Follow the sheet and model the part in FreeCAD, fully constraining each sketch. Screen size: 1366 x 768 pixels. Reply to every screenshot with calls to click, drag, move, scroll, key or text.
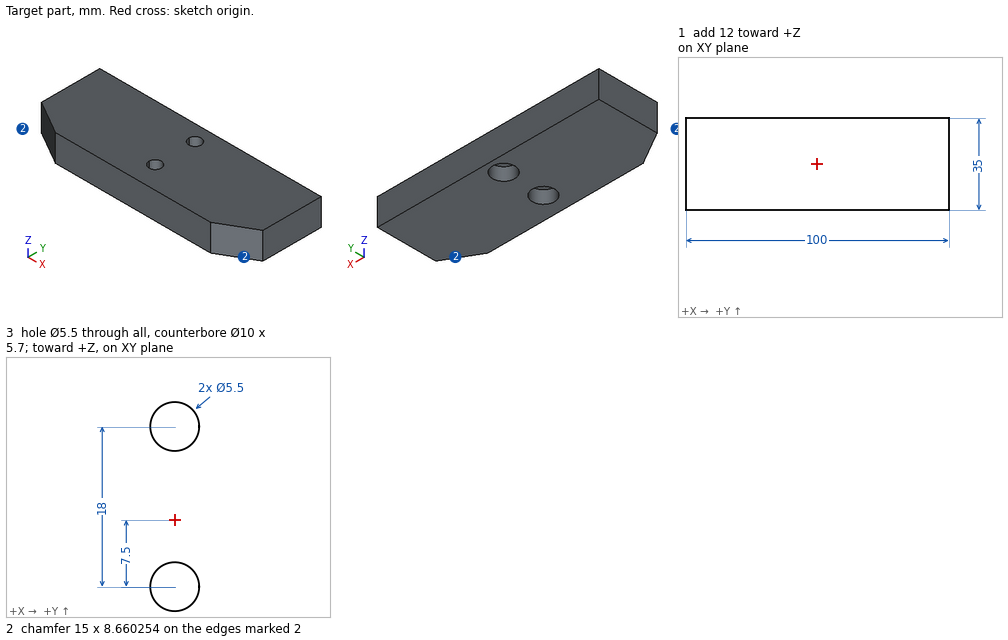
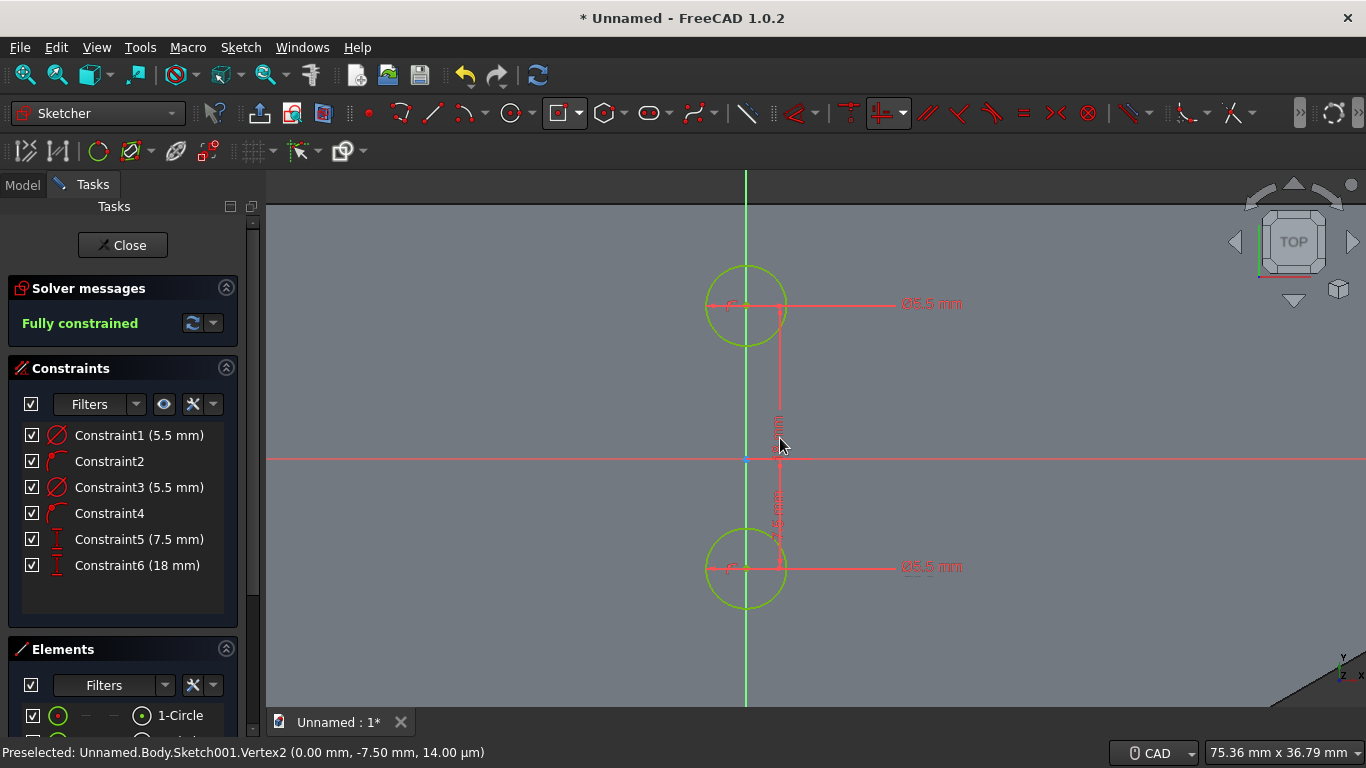
click(123, 245)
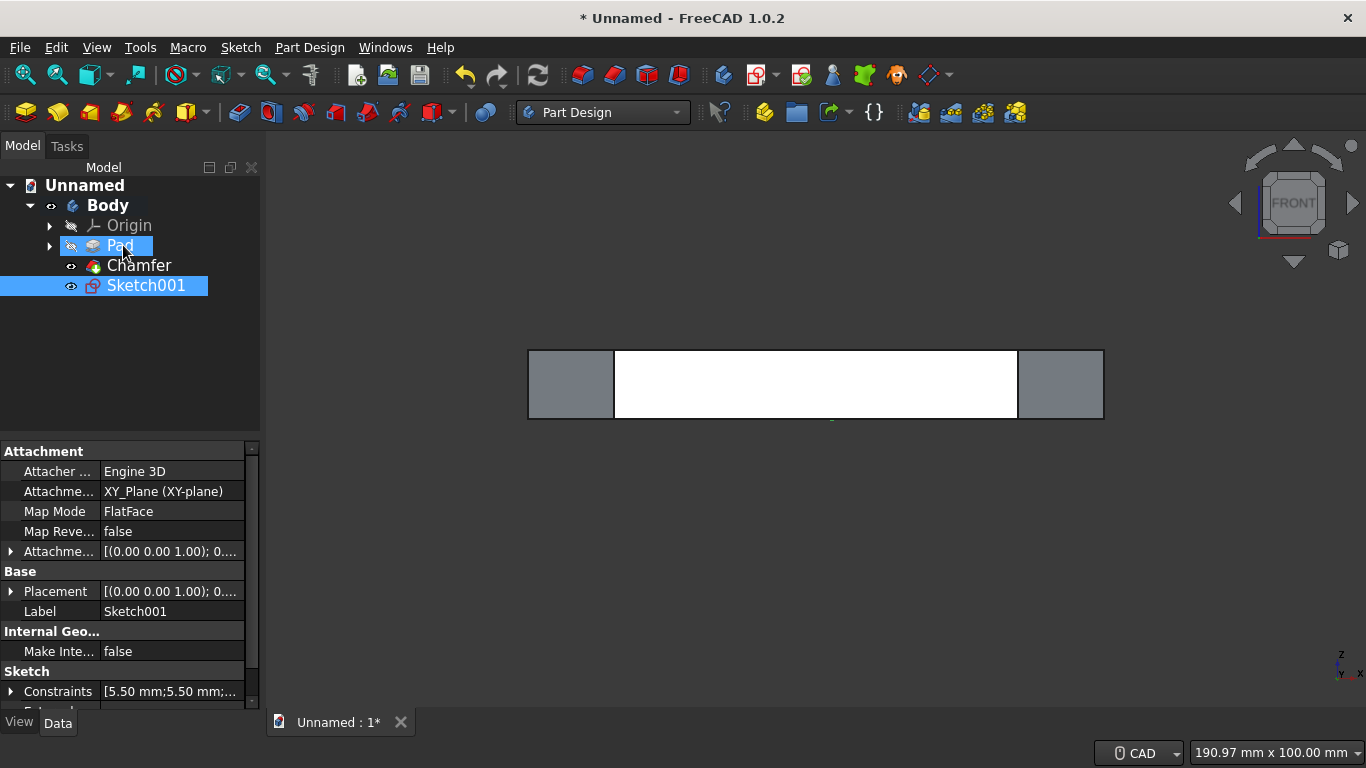
click(272, 112)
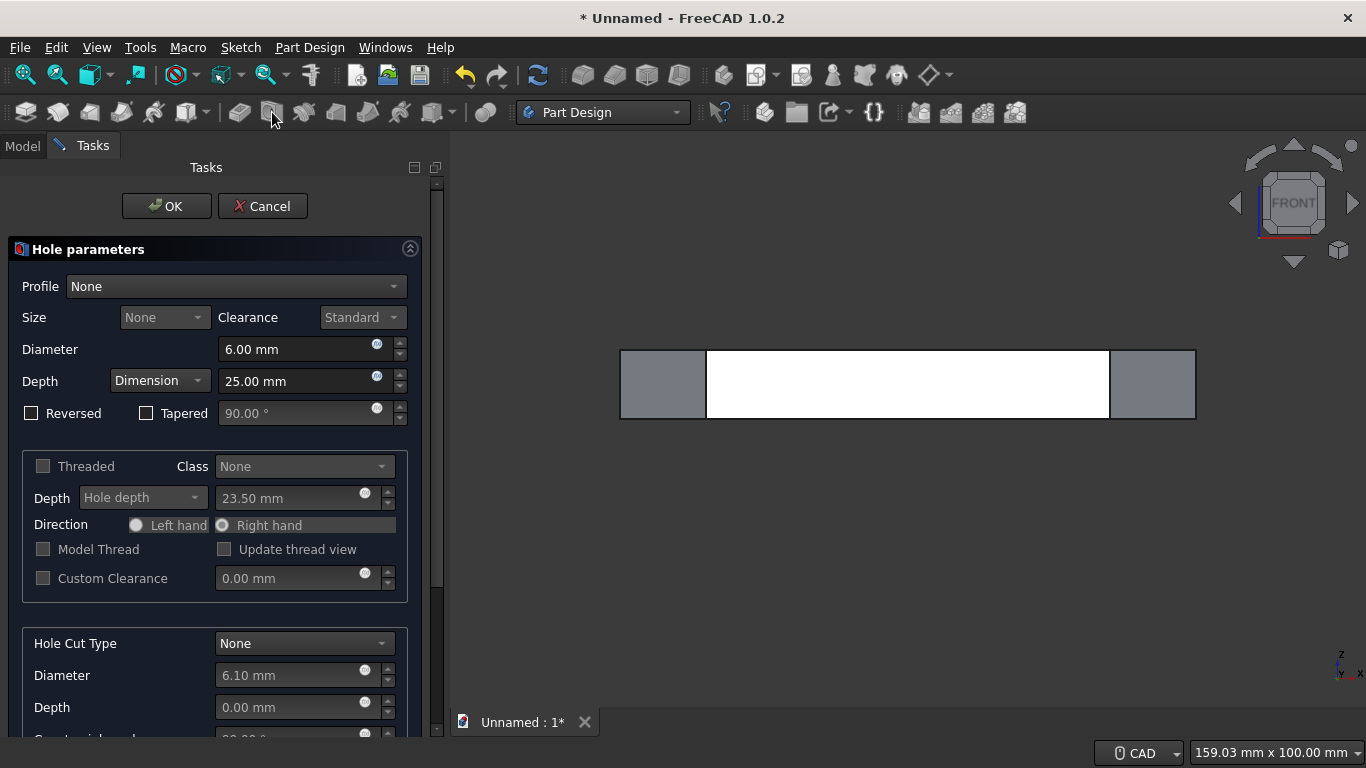
triple_click(305, 349)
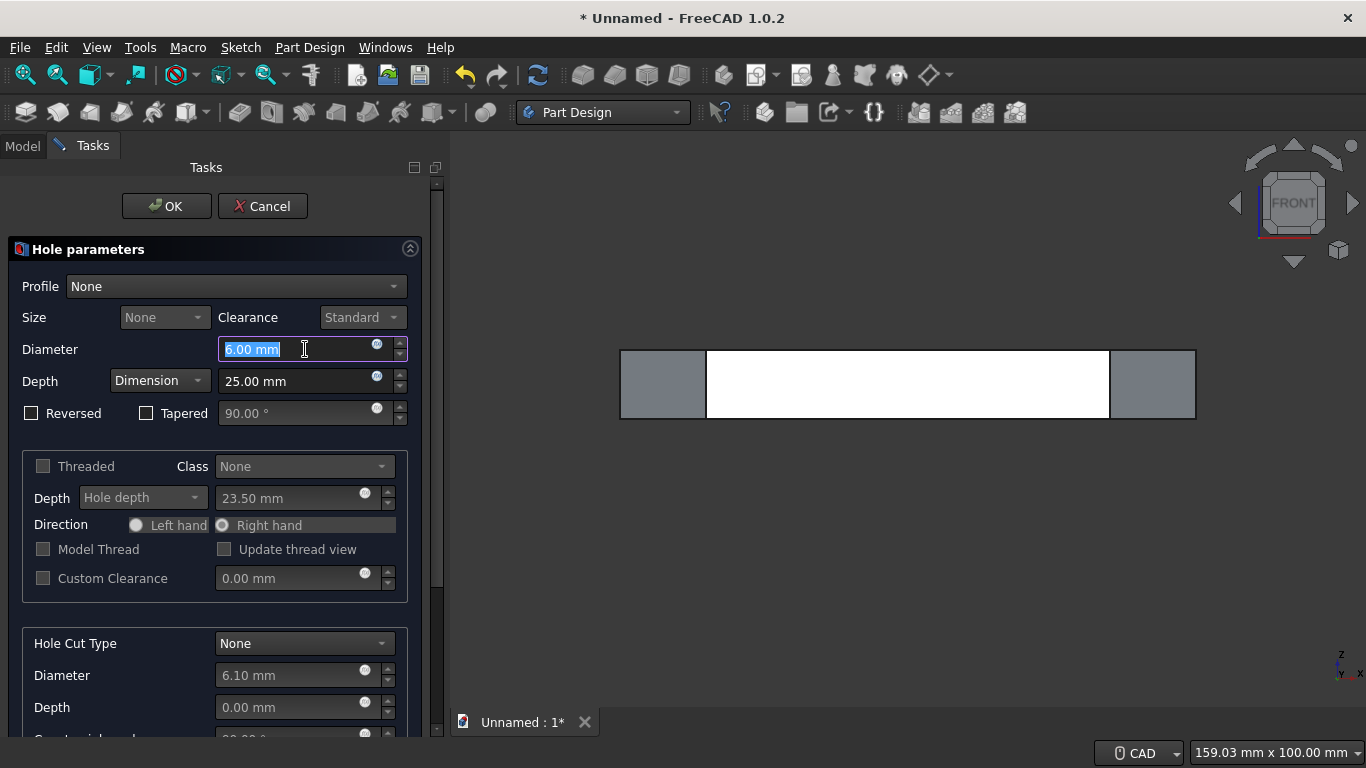
text(5.5)
key(Tab)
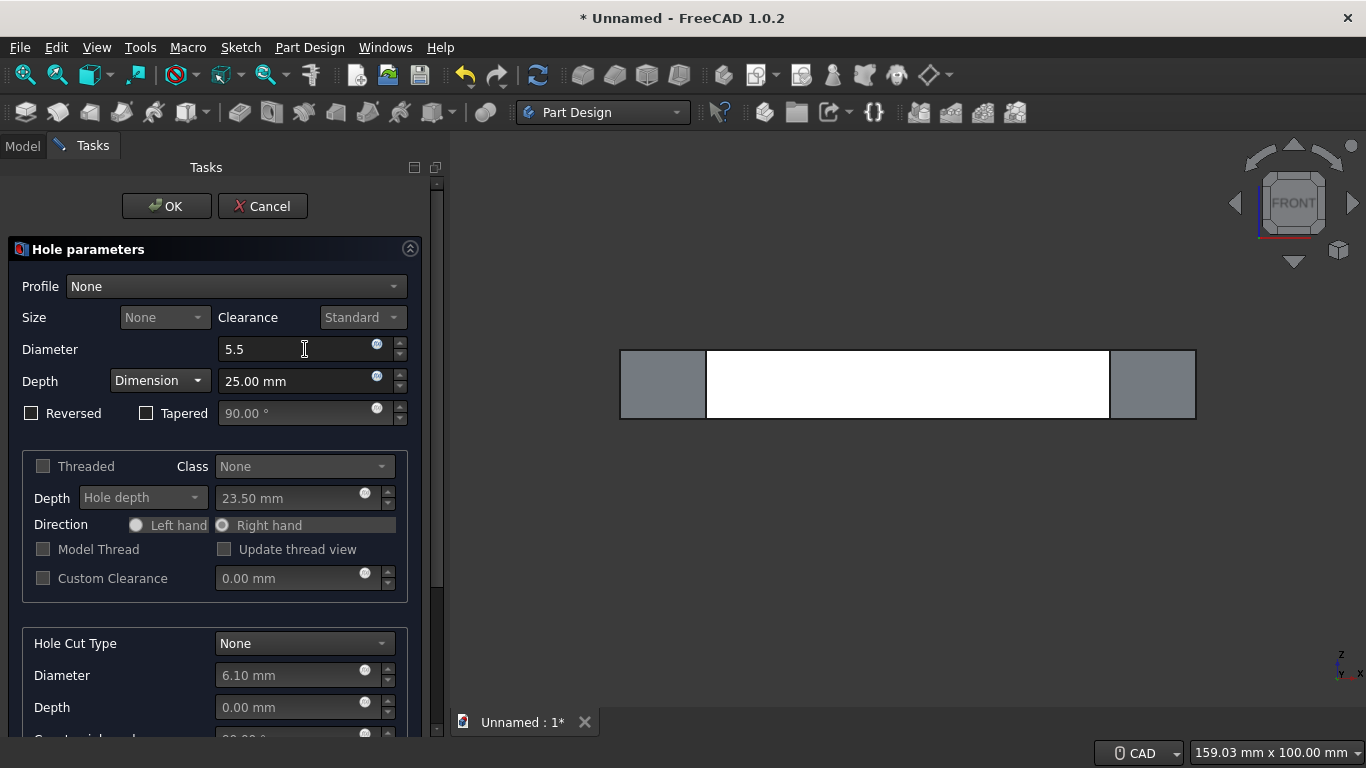
click(161, 380)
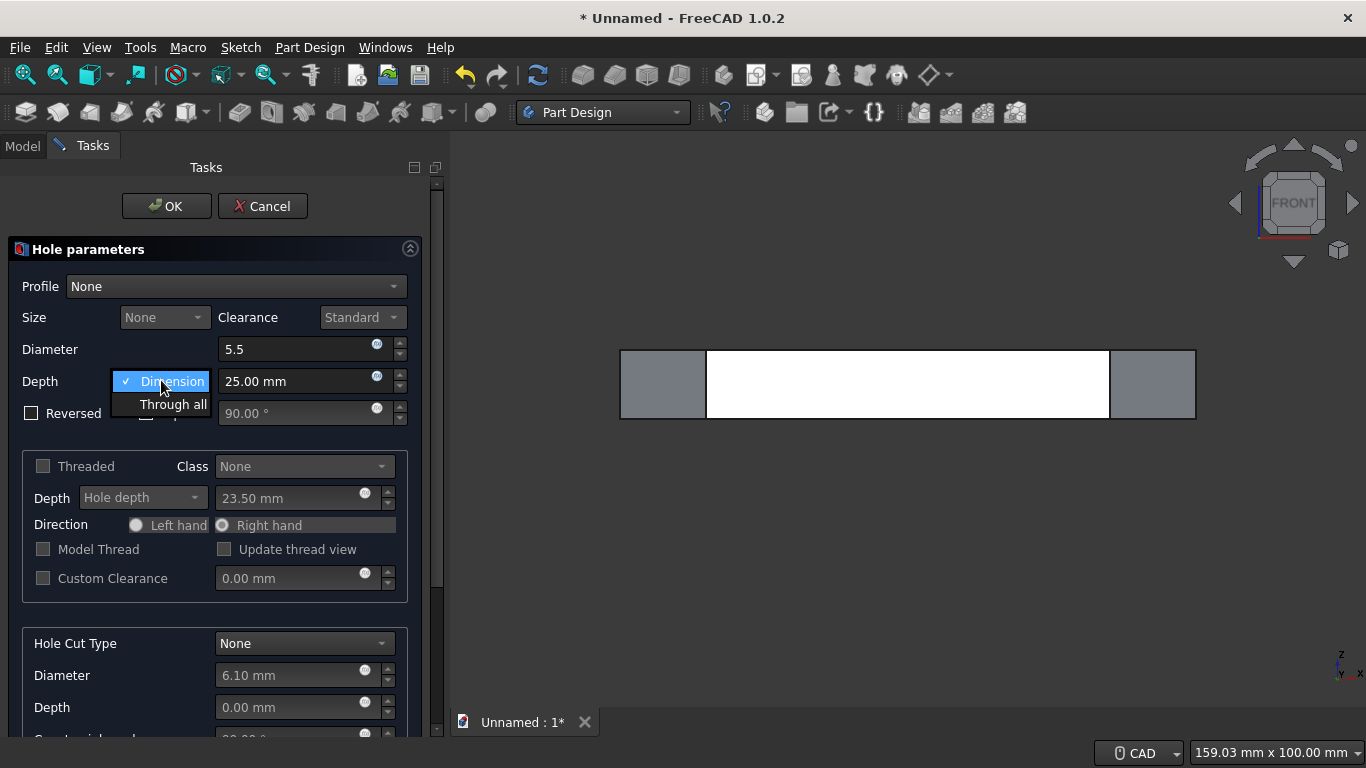
click(160, 404)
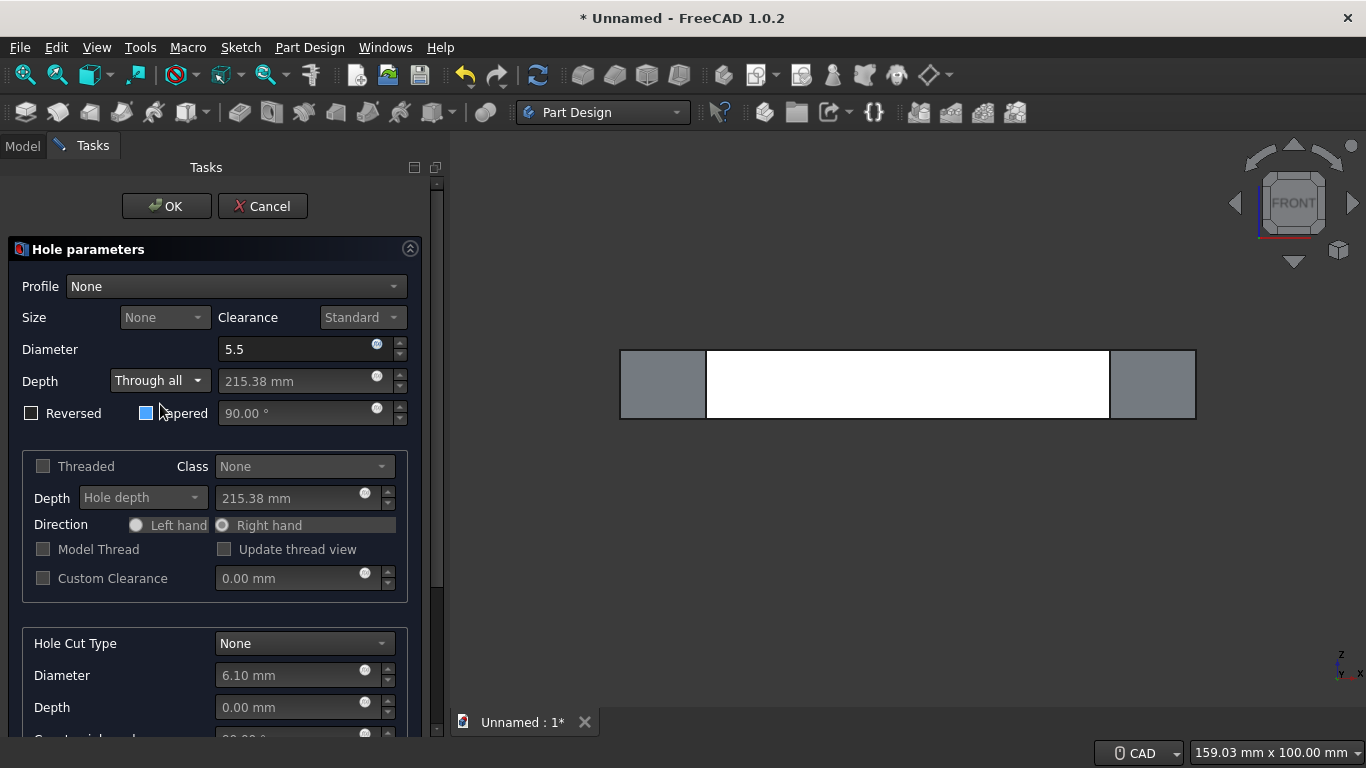
click(30, 413)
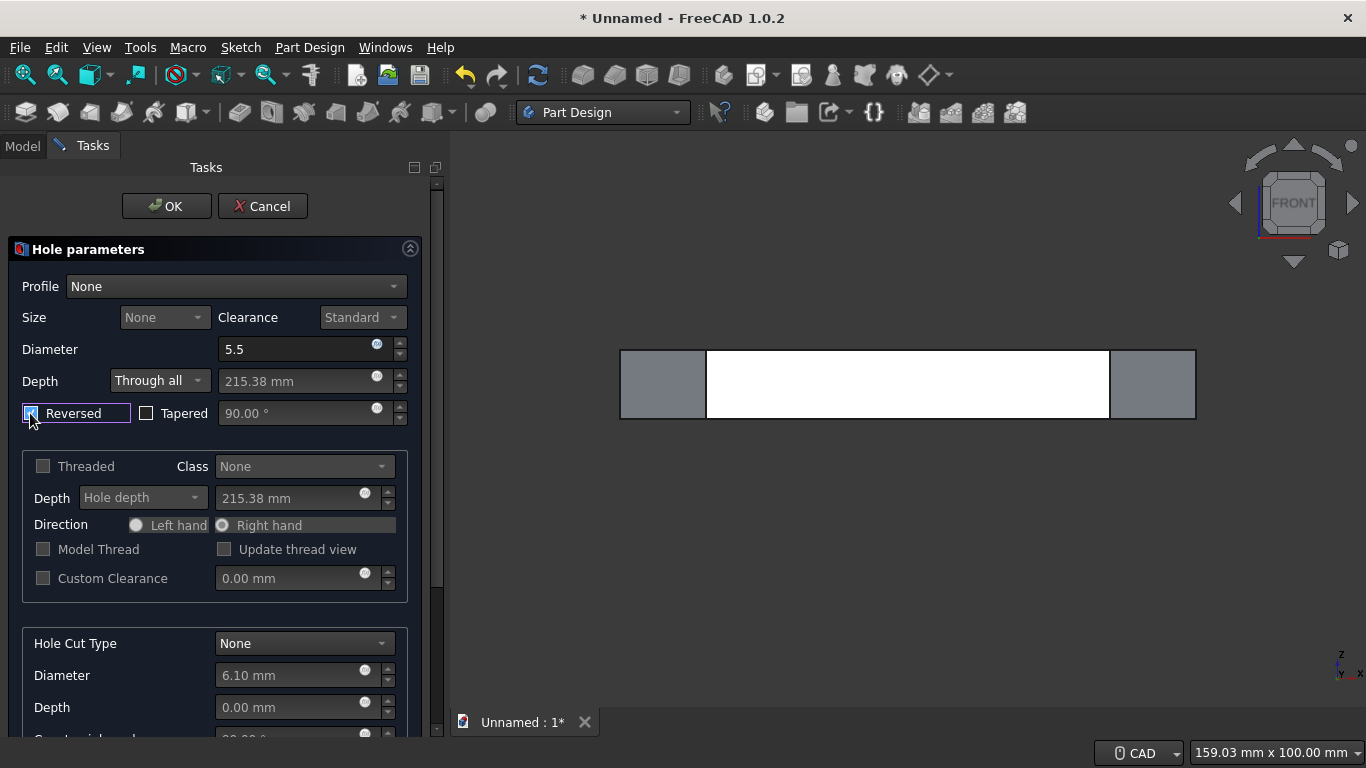
click(306, 644)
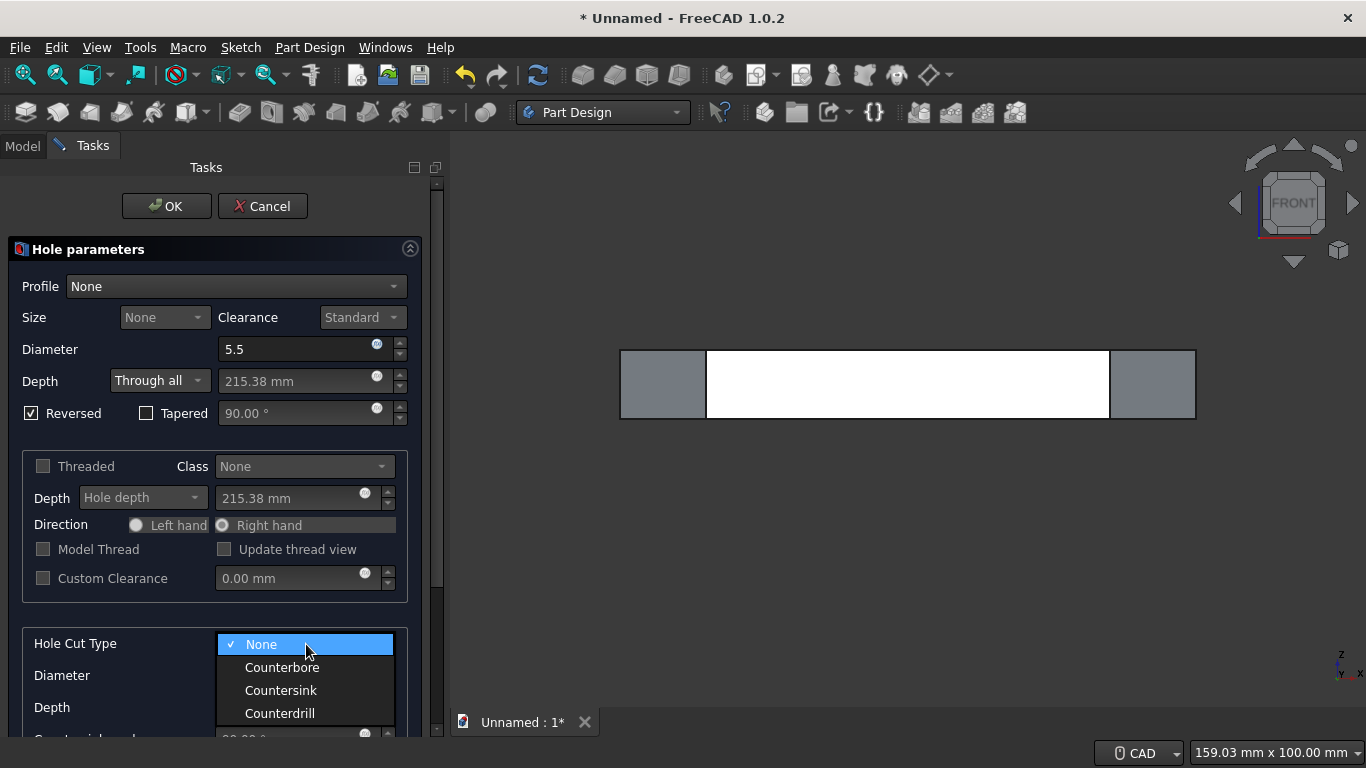
click(304, 668)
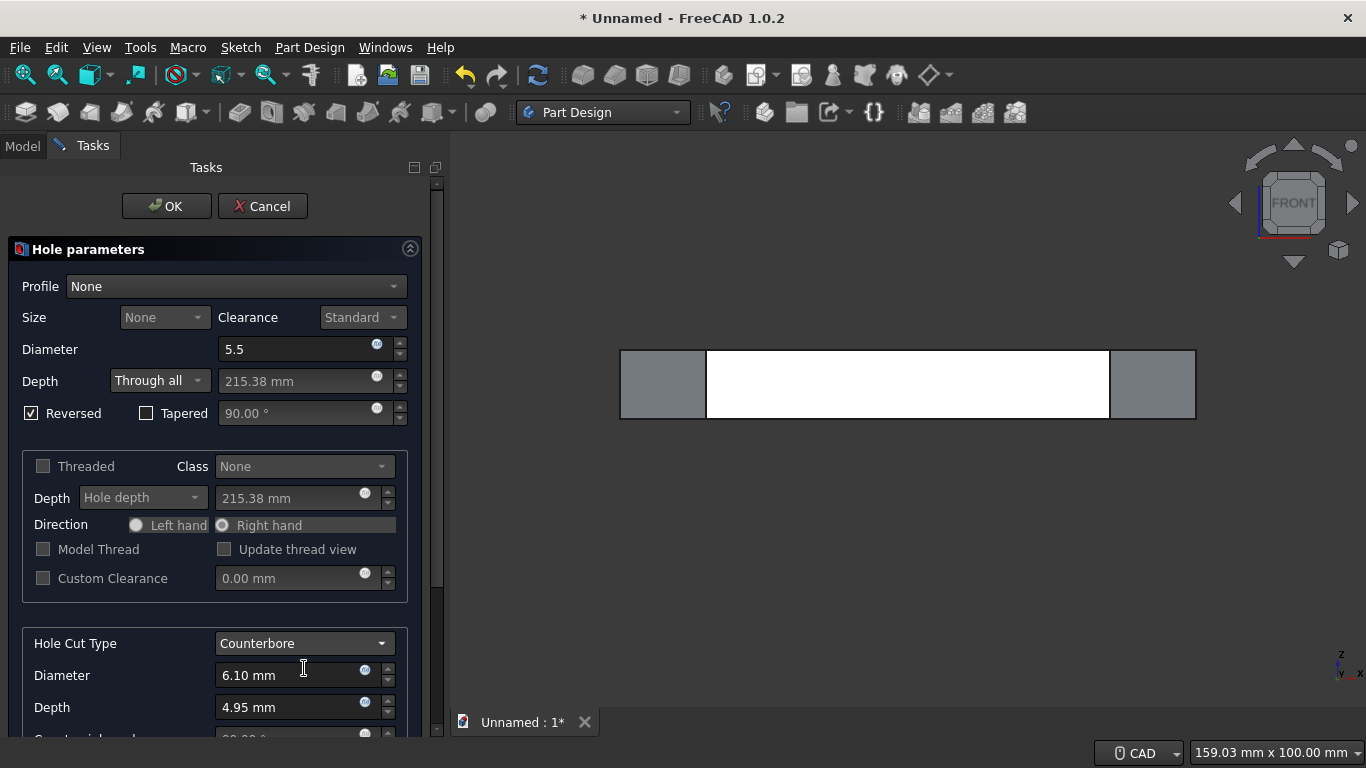
triple_click(298, 675)